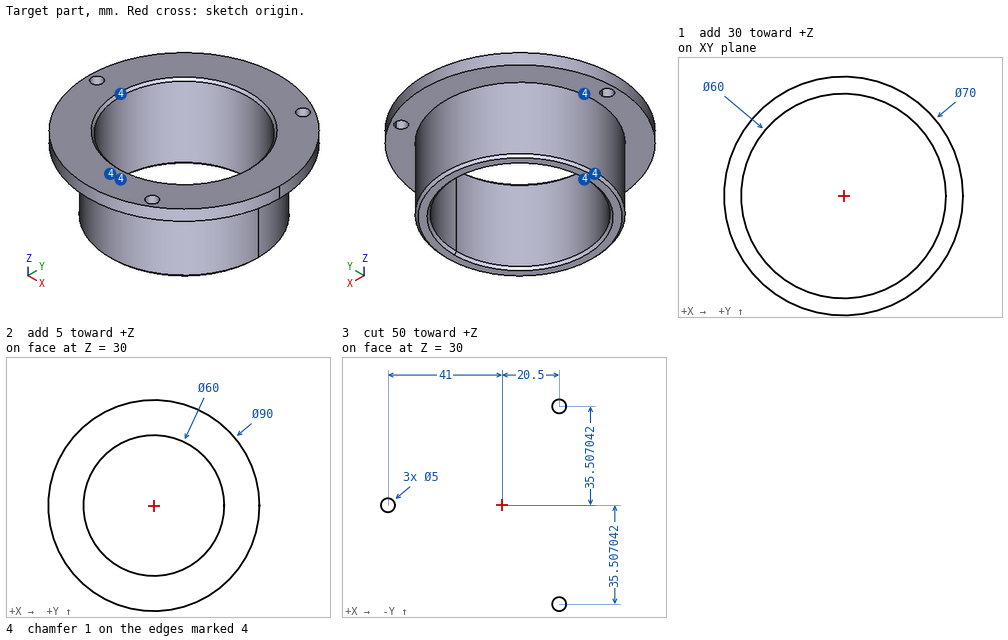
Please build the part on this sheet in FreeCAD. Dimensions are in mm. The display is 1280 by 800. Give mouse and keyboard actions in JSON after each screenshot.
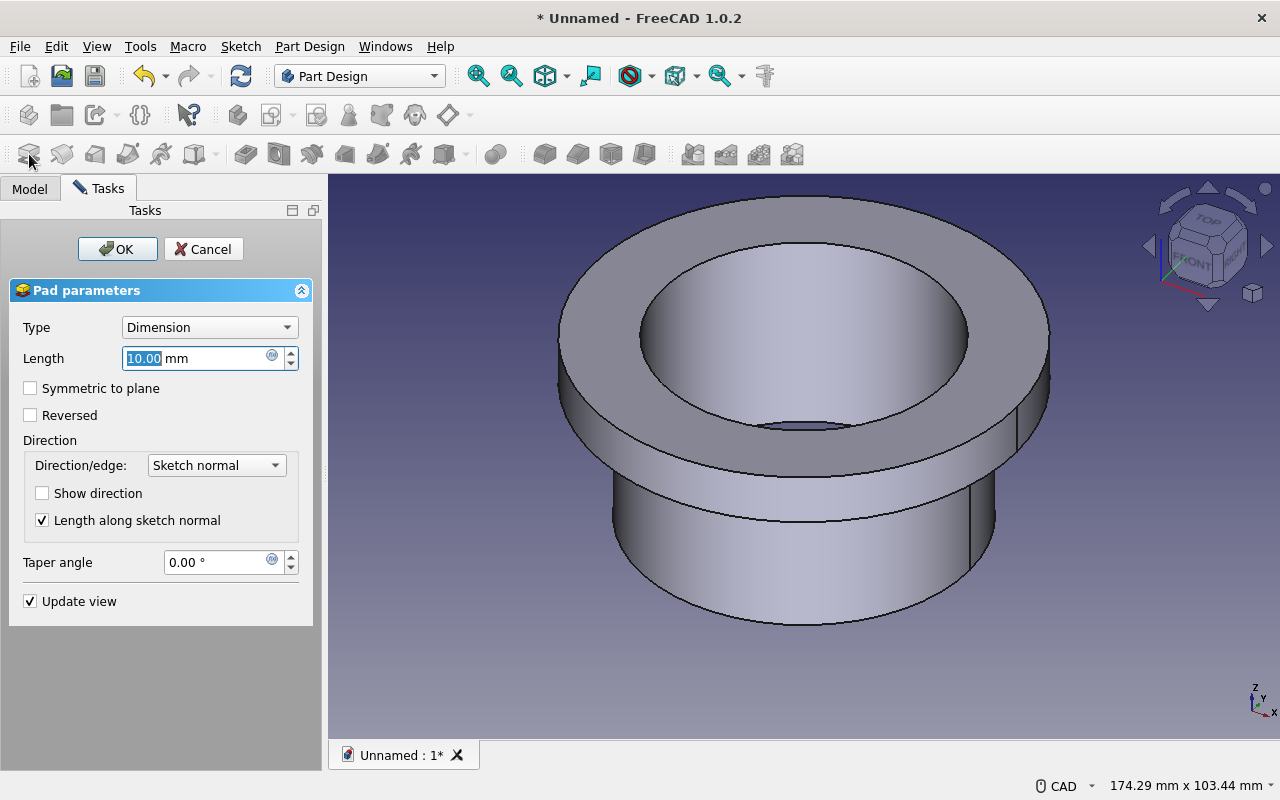
{"action": "type", "text": "5"}
{"action": "key", "text": "Tab"}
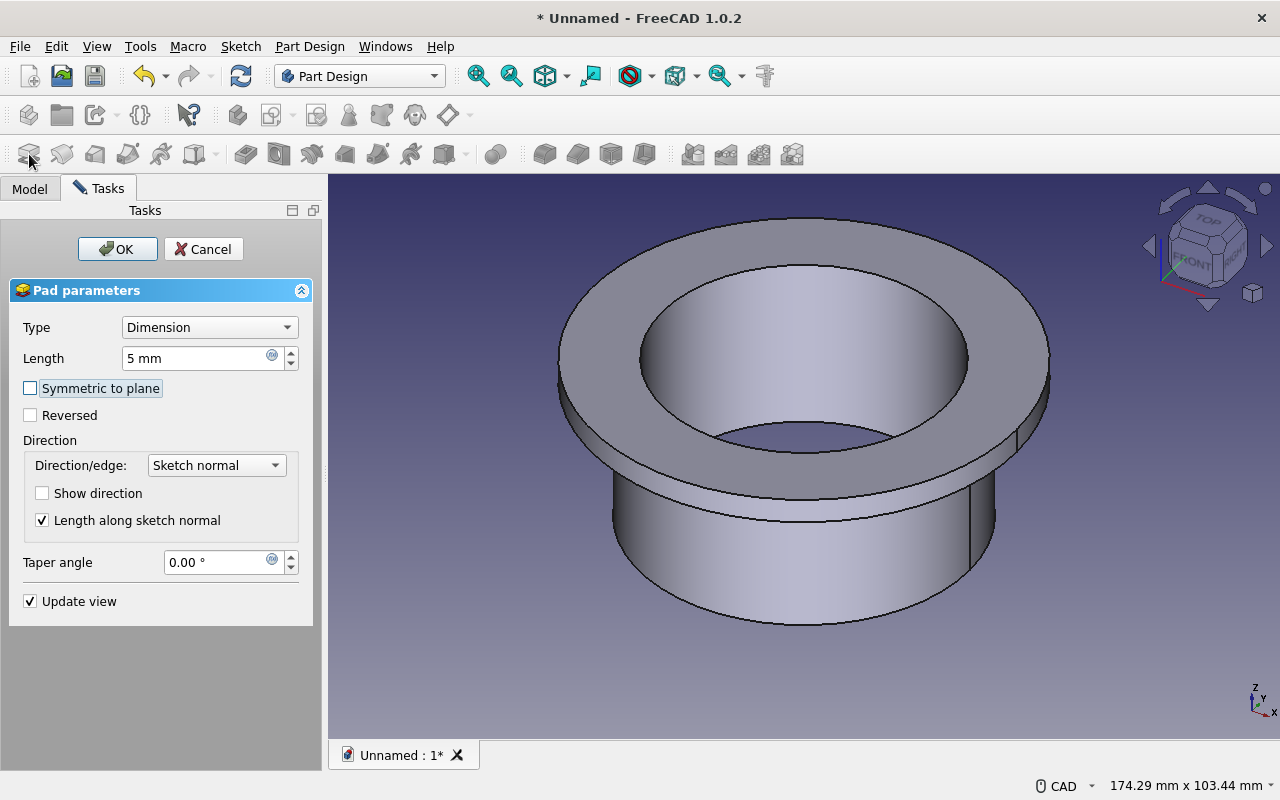
{"action": "left_click", "coordinate": [118, 249]}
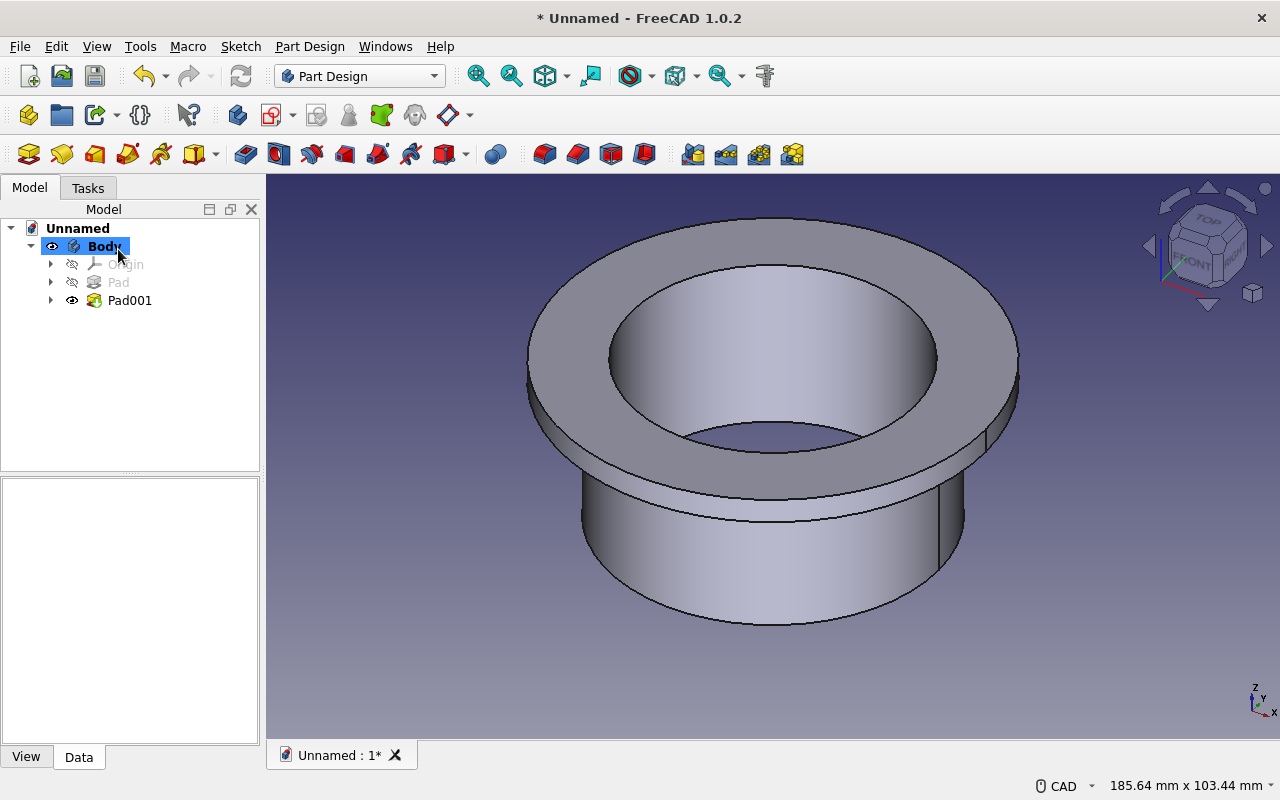
{"action": "left_click", "coordinate": [479, 76]}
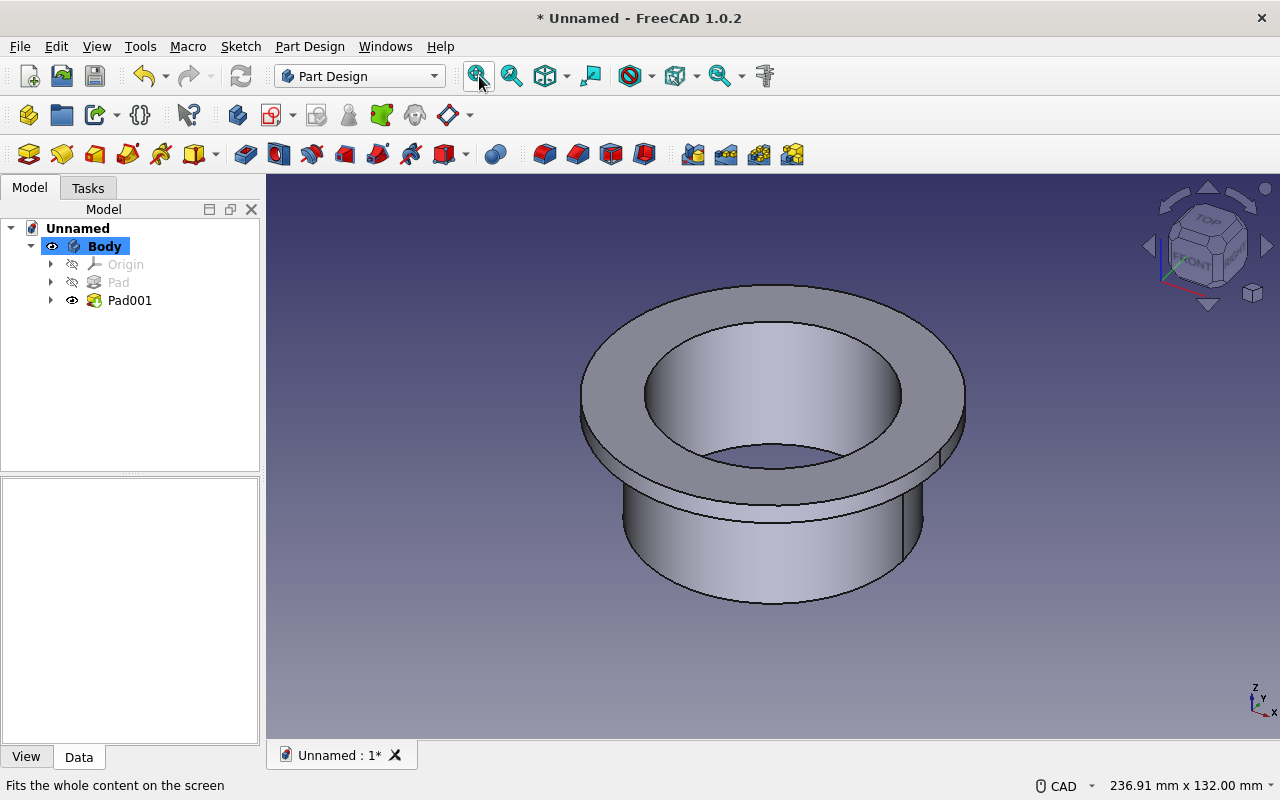
{"action": "key", "text": "5"}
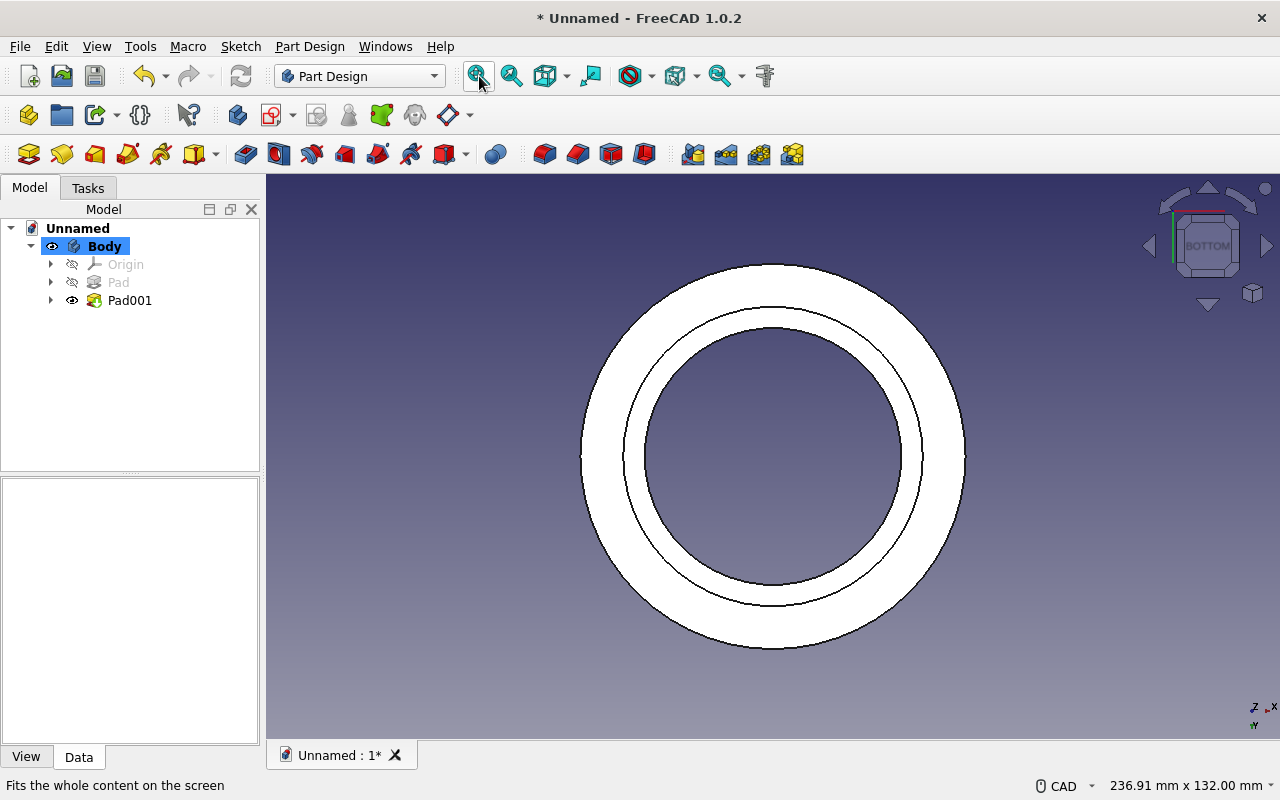
{"action": "left_click", "coordinate": [608, 400]}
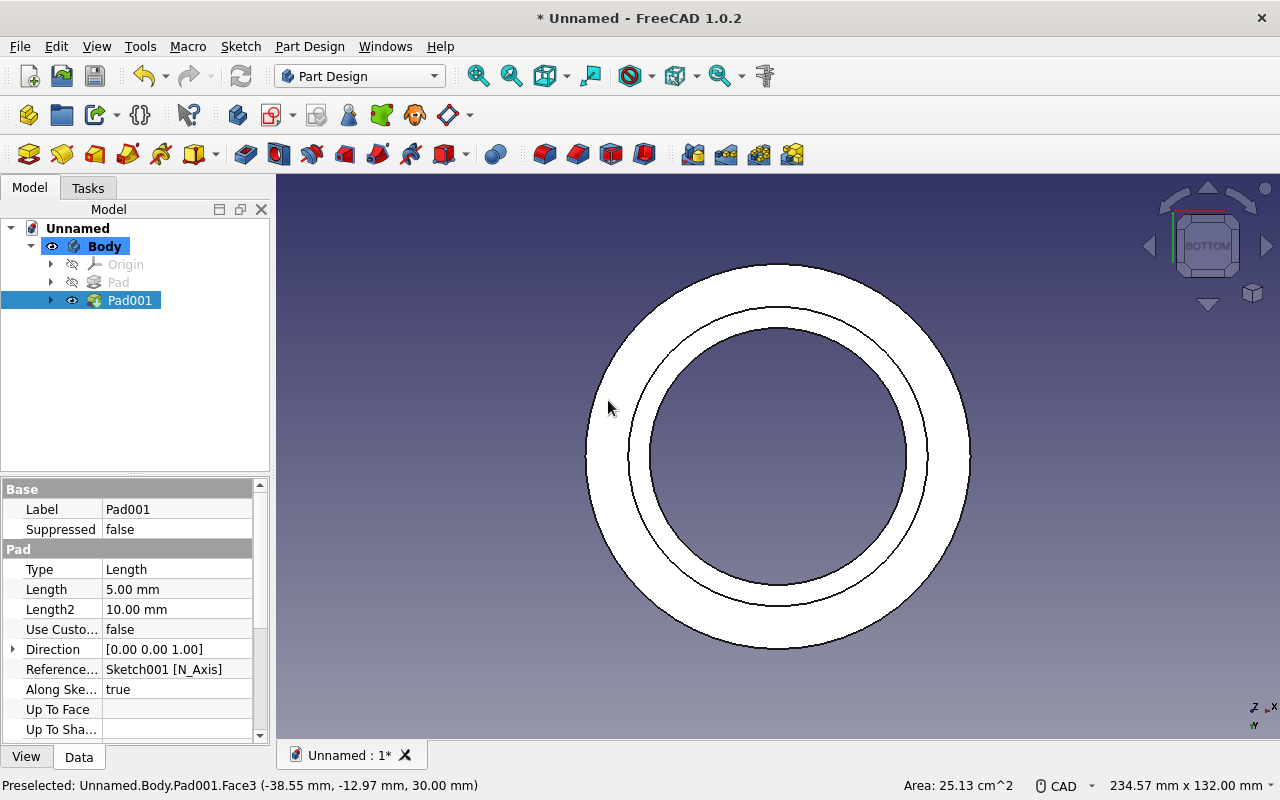
{"action": "left_click", "coordinate": [270, 116]}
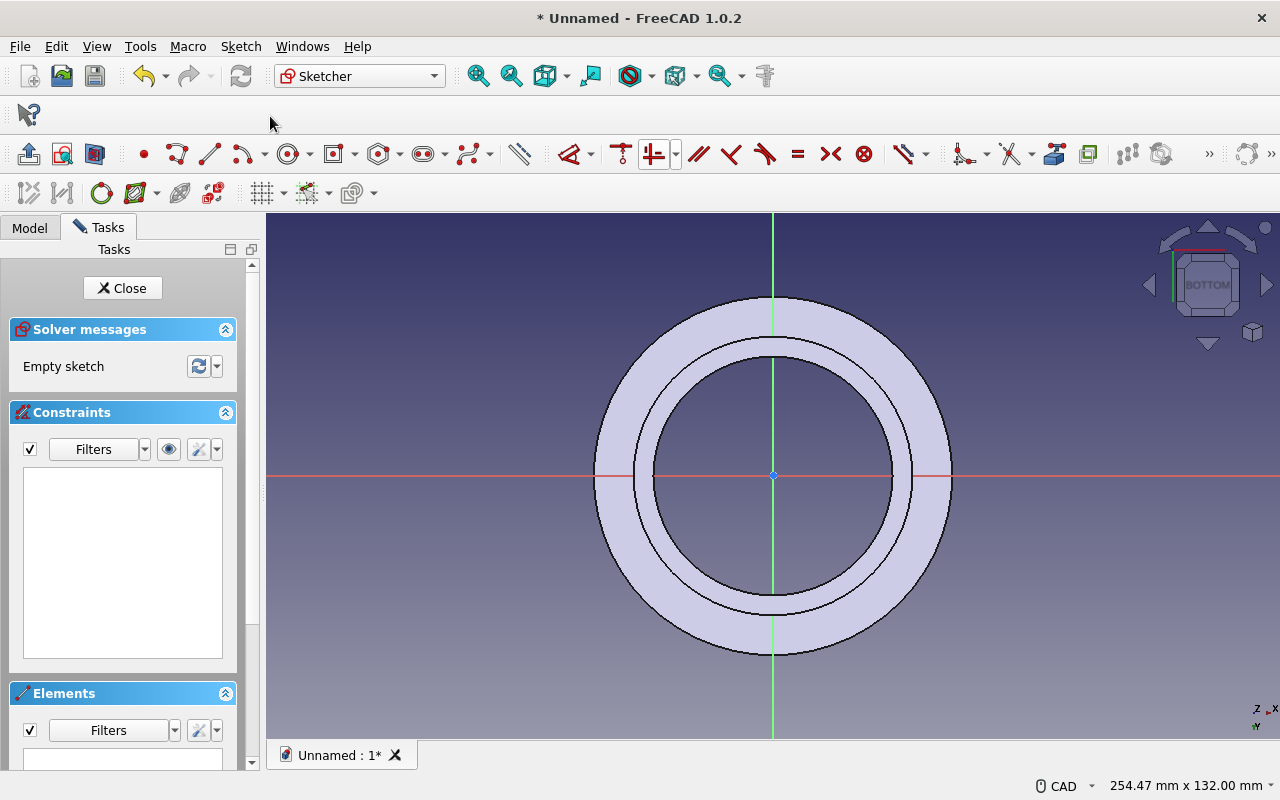
{"action": "key", "text": "g c"}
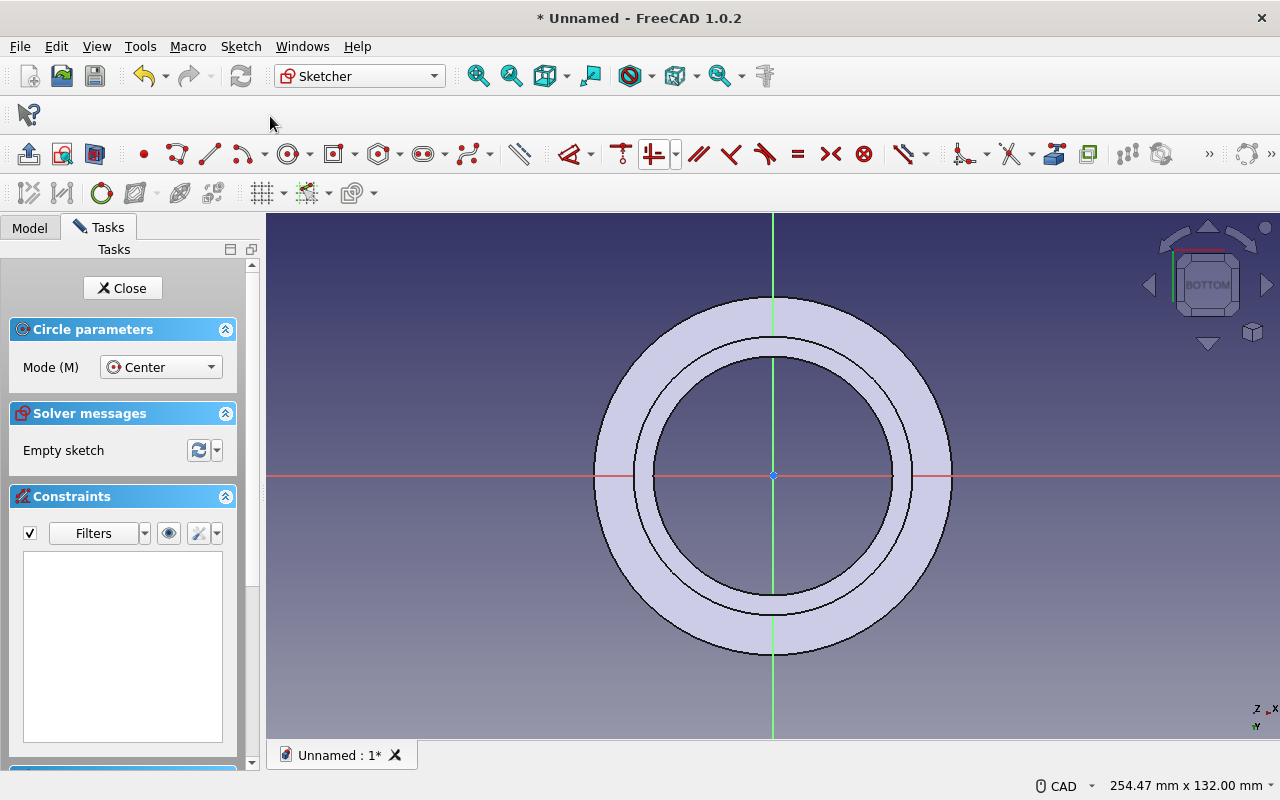
{"action": "scroll", "coordinate": [610, 476], "scroll_direction": "up", "scroll_amount": 5}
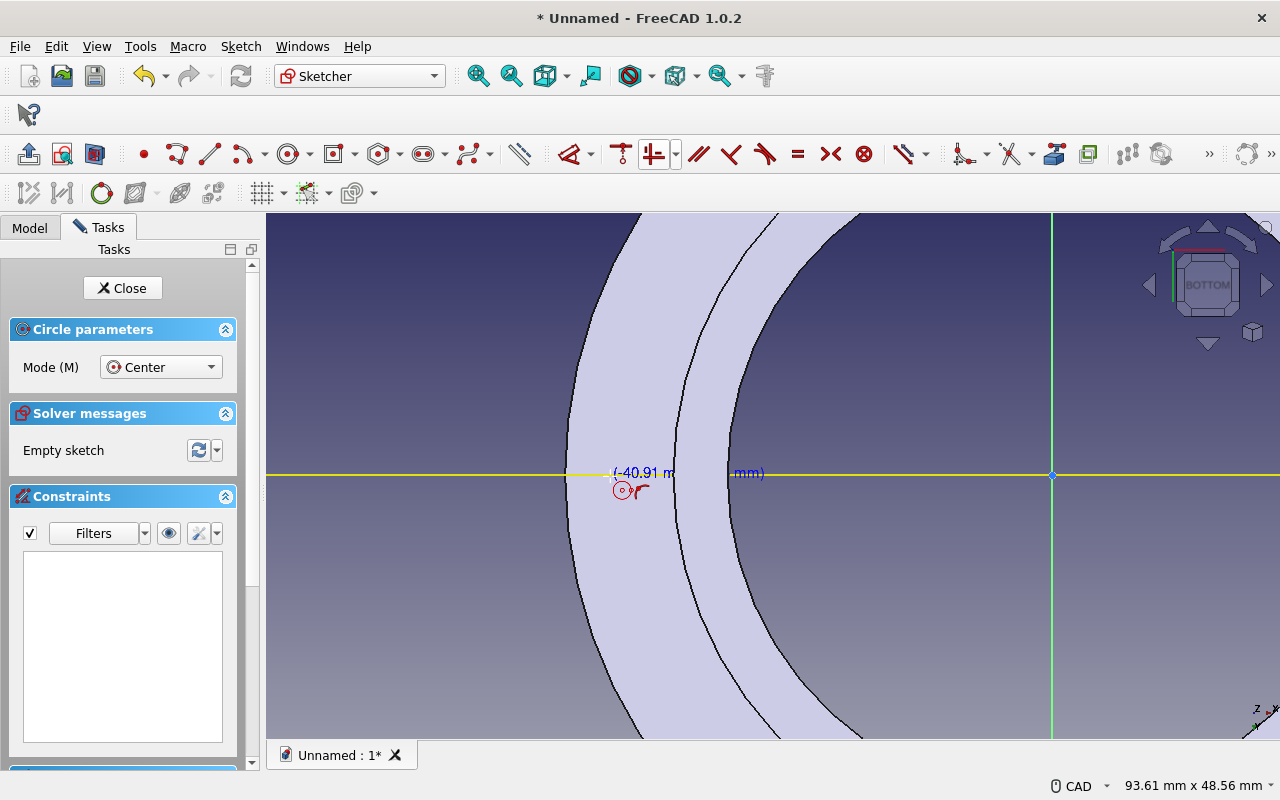
{"action": "left_click", "coordinate": [608, 475]}
{"action": "left_click", "coordinate": [628, 456]}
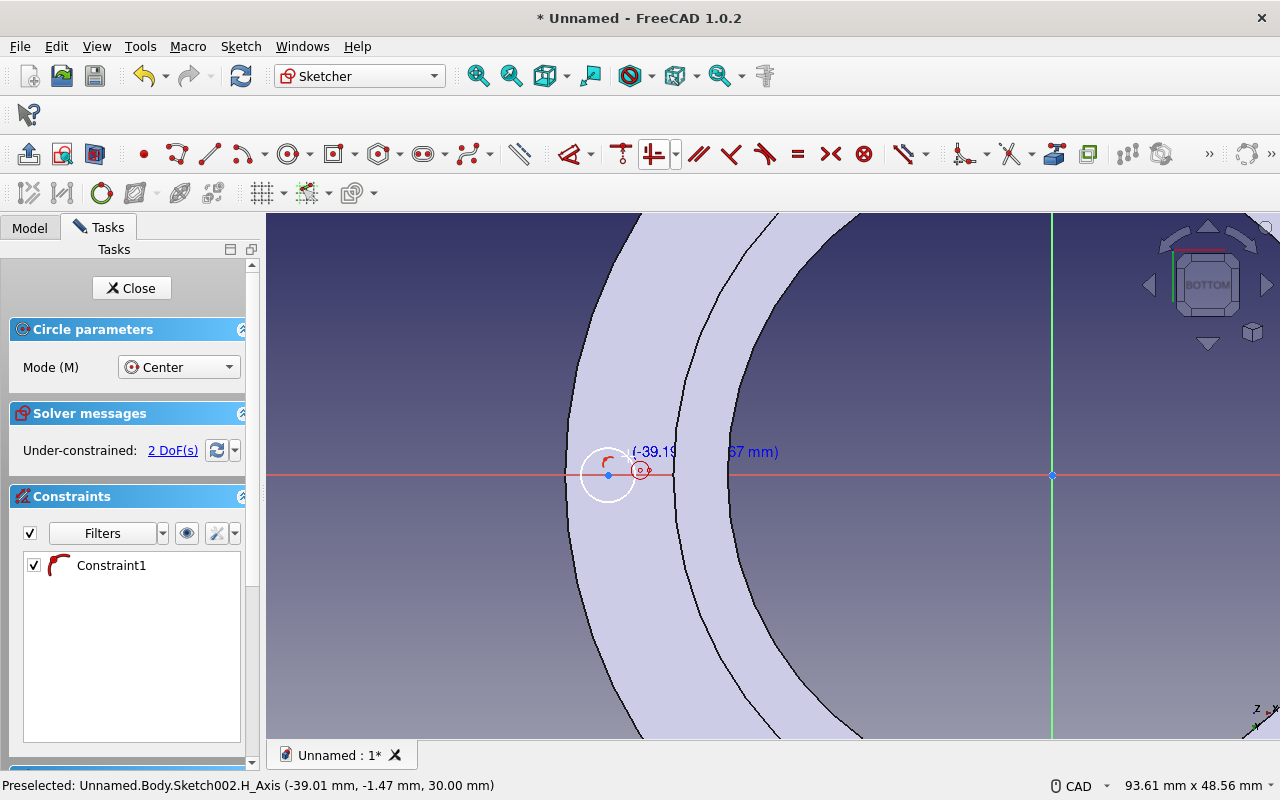
{"action": "scroll", "coordinate": [567, 477], "scroll_direction": "down", "scroll_amount": 5}